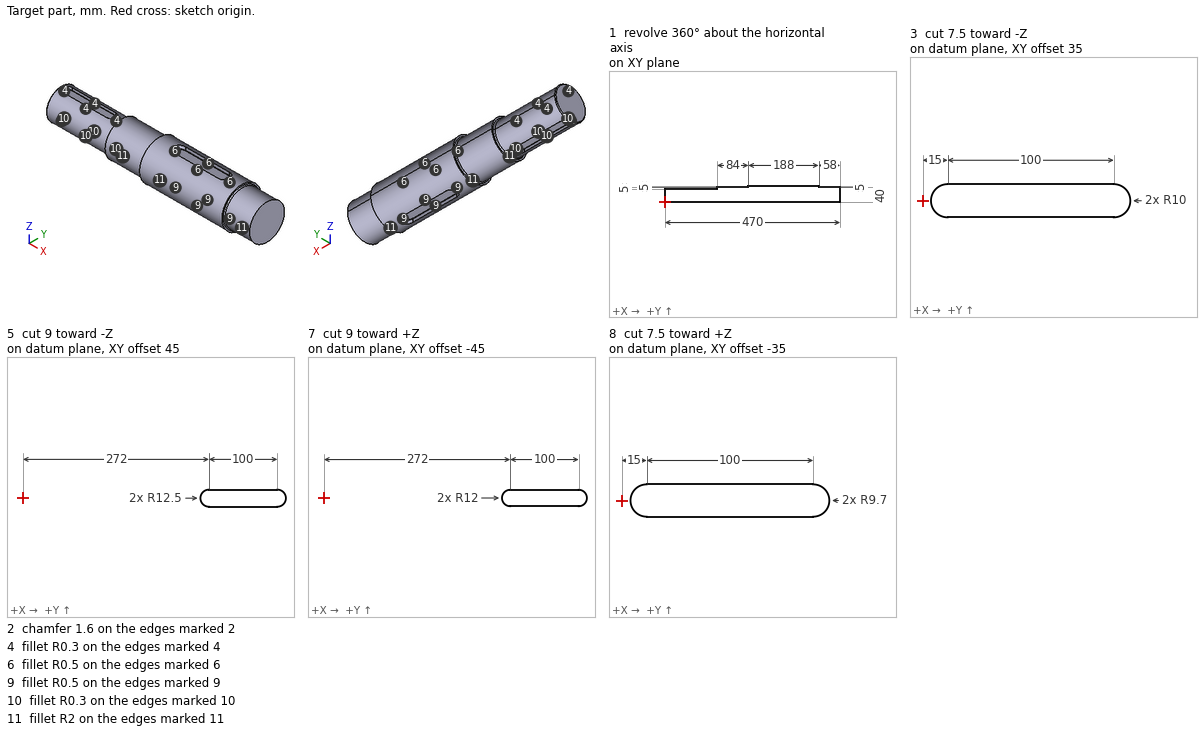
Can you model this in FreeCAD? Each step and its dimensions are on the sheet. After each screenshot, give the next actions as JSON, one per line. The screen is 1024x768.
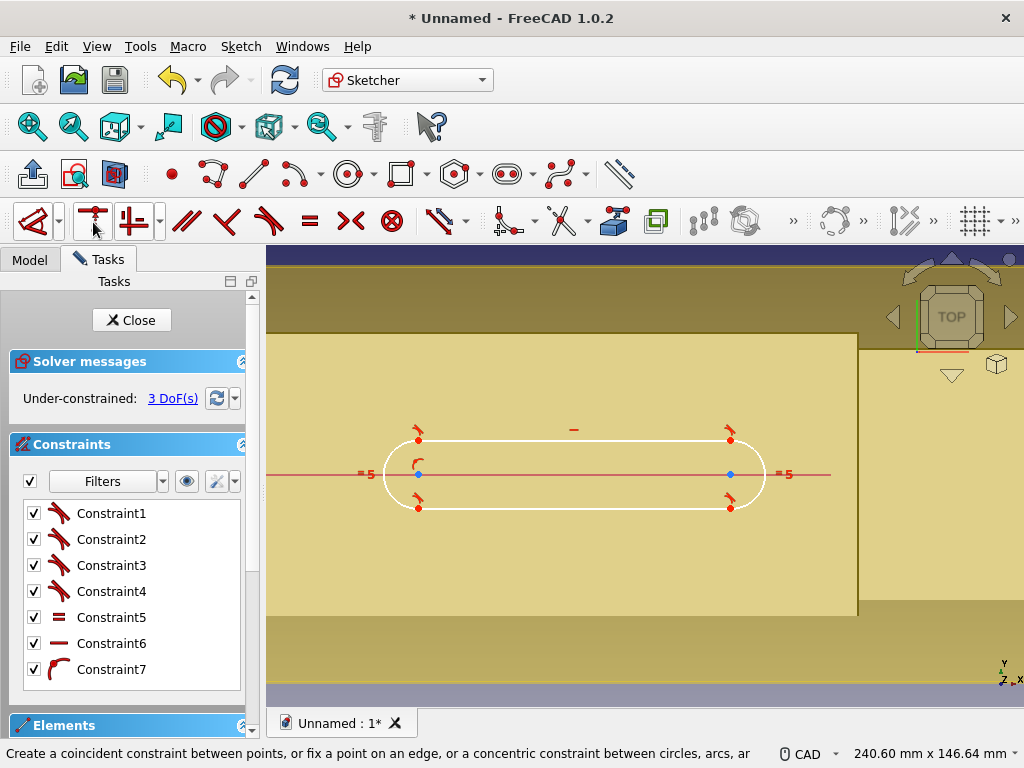
{"action": "left_click", "coordinate": [390, 455]}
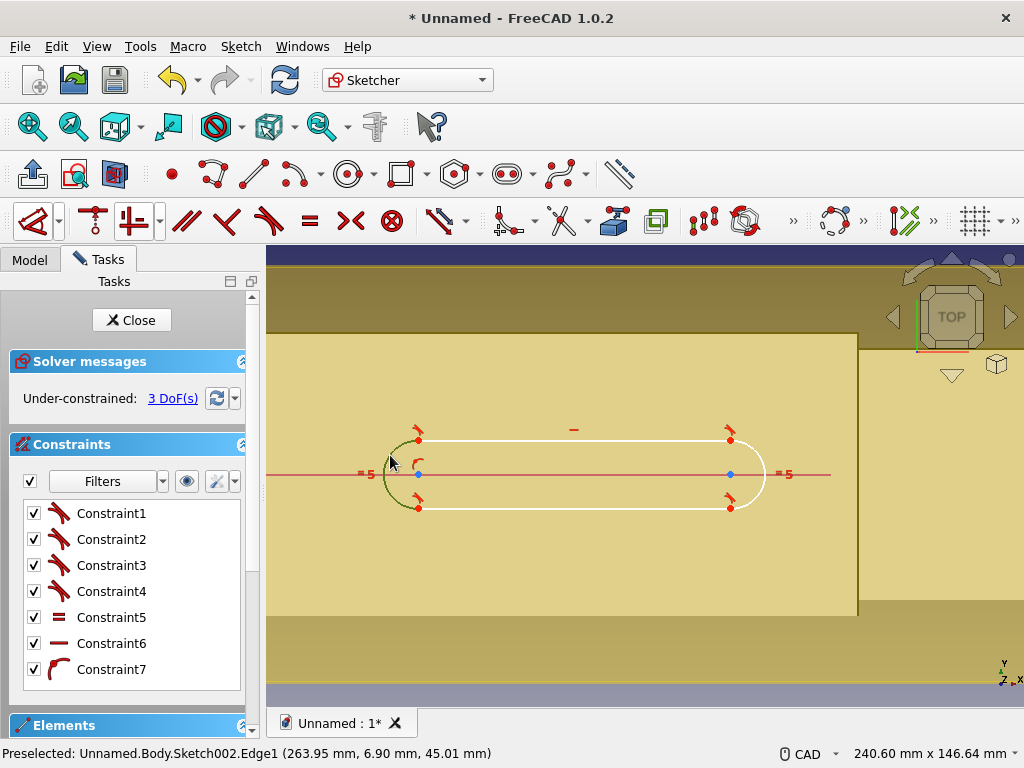
{"action": "left_click", "coordinate": [58, 222]}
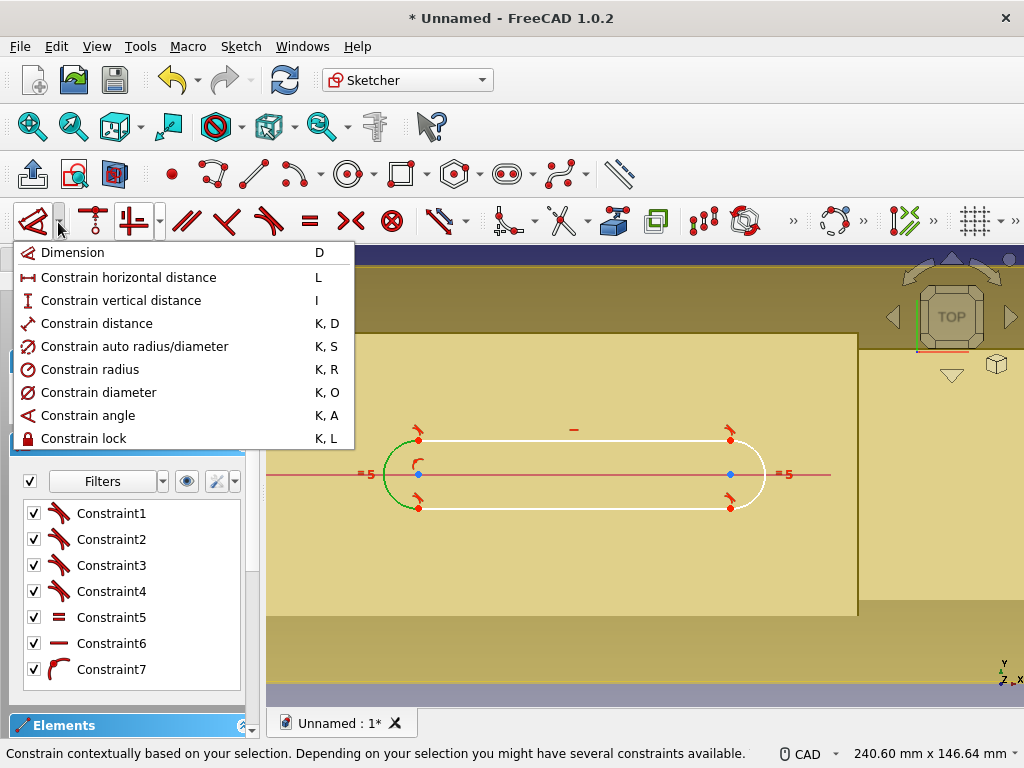
{"action": "left_click", "coordinate": [184, 370]}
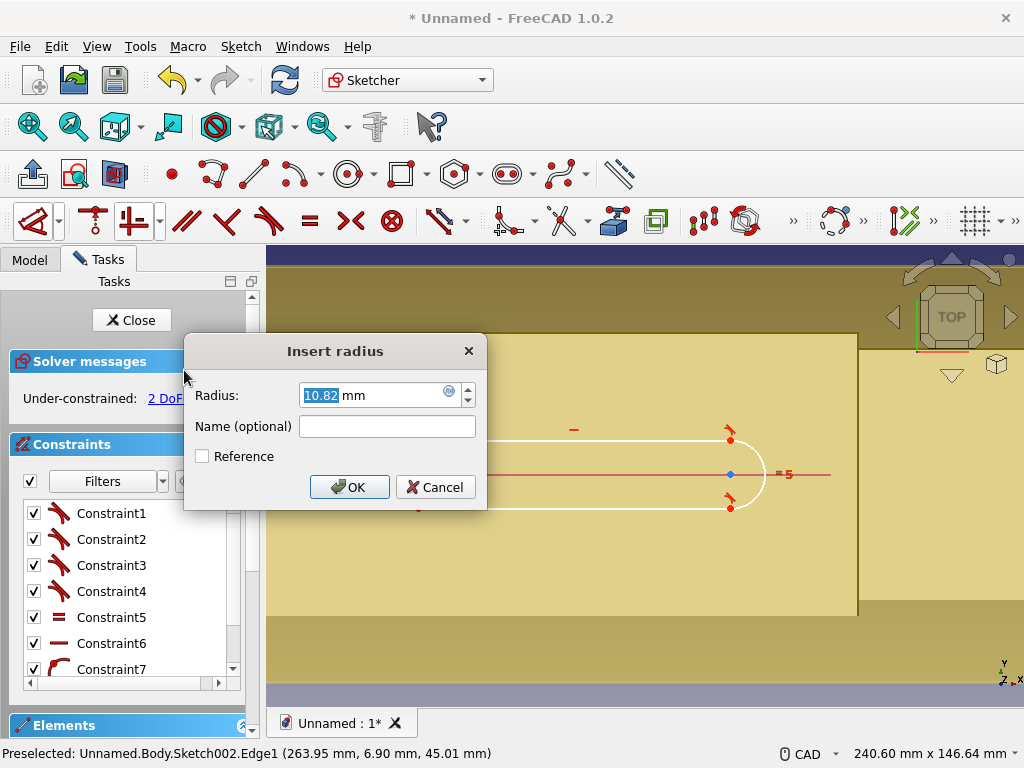
{"action": "type", "text": "12.5"}
{"action": "key", "text": "Return"}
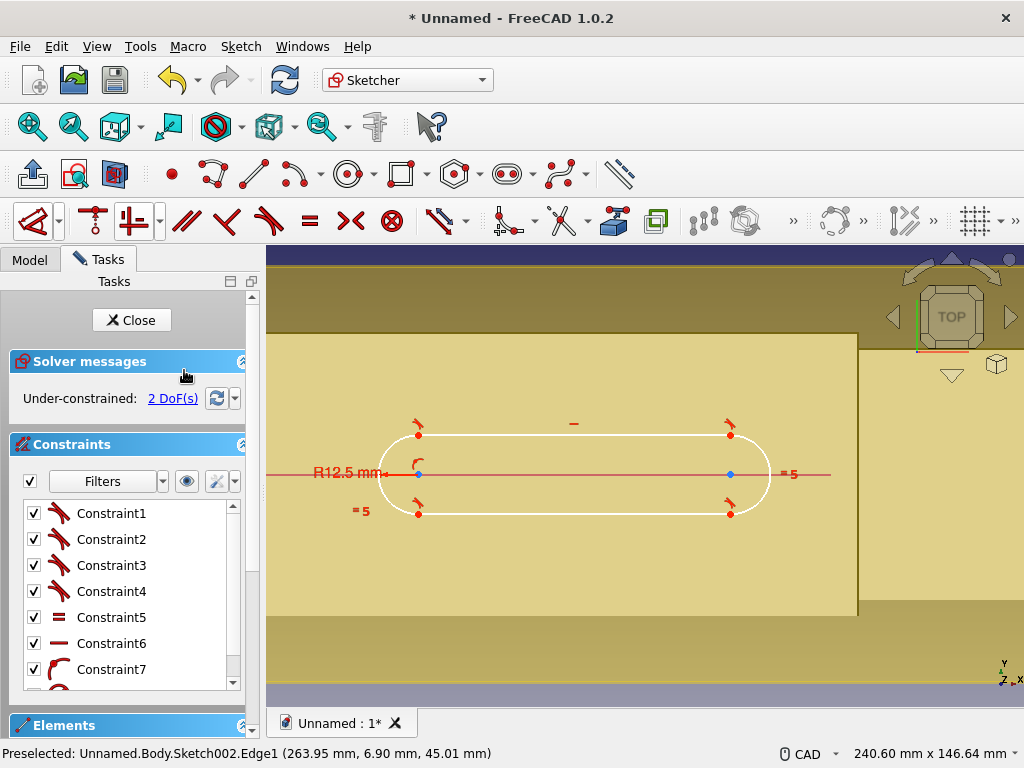
{"action": "left_click", "coordinate": [512, 435]}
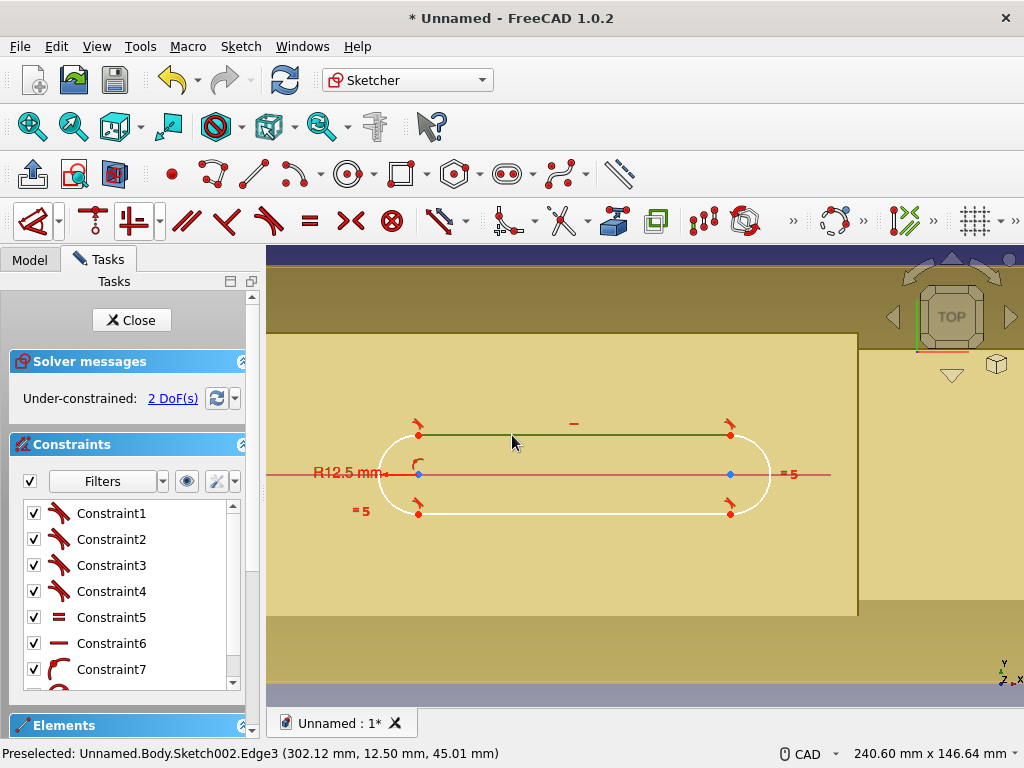
{"action": "key", "text": "l"}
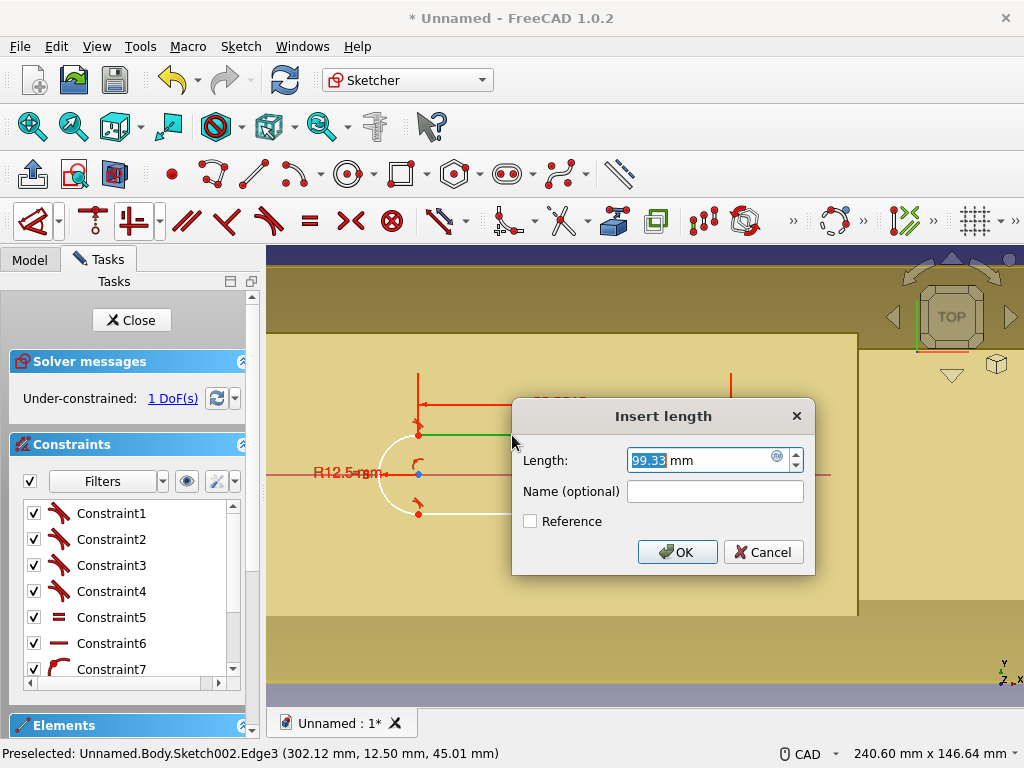
{"action": "type", "text": "100"}
{"action": "key", "text": "Return"}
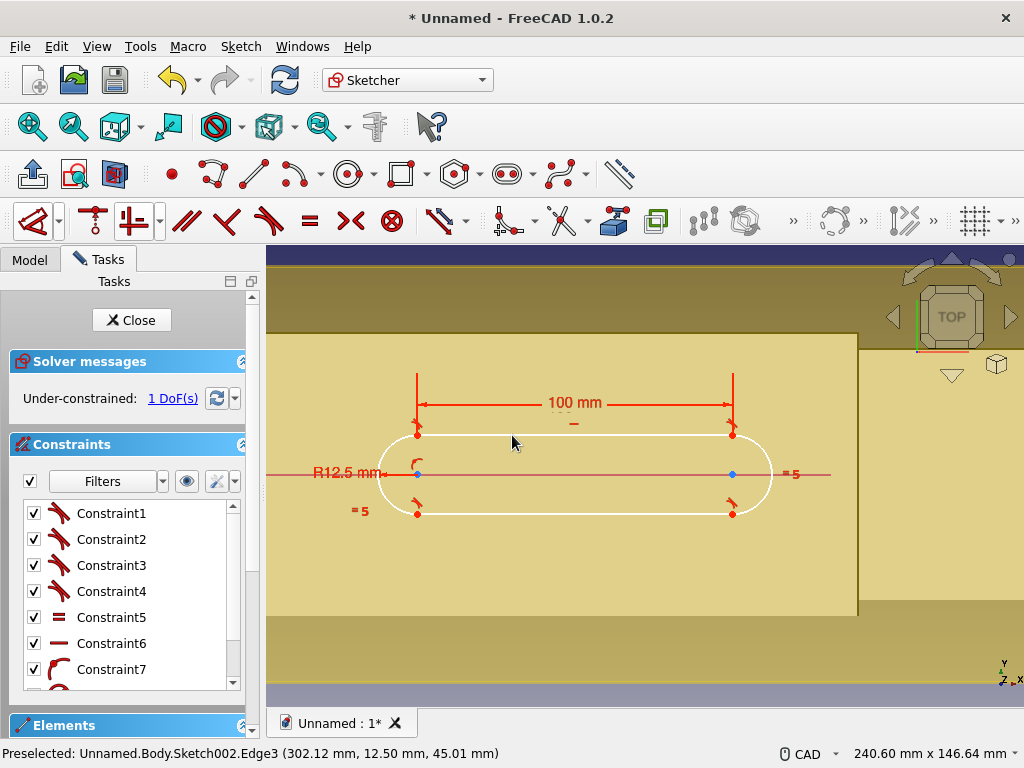
{"action": "left_click", "coordinate": [417, 435]}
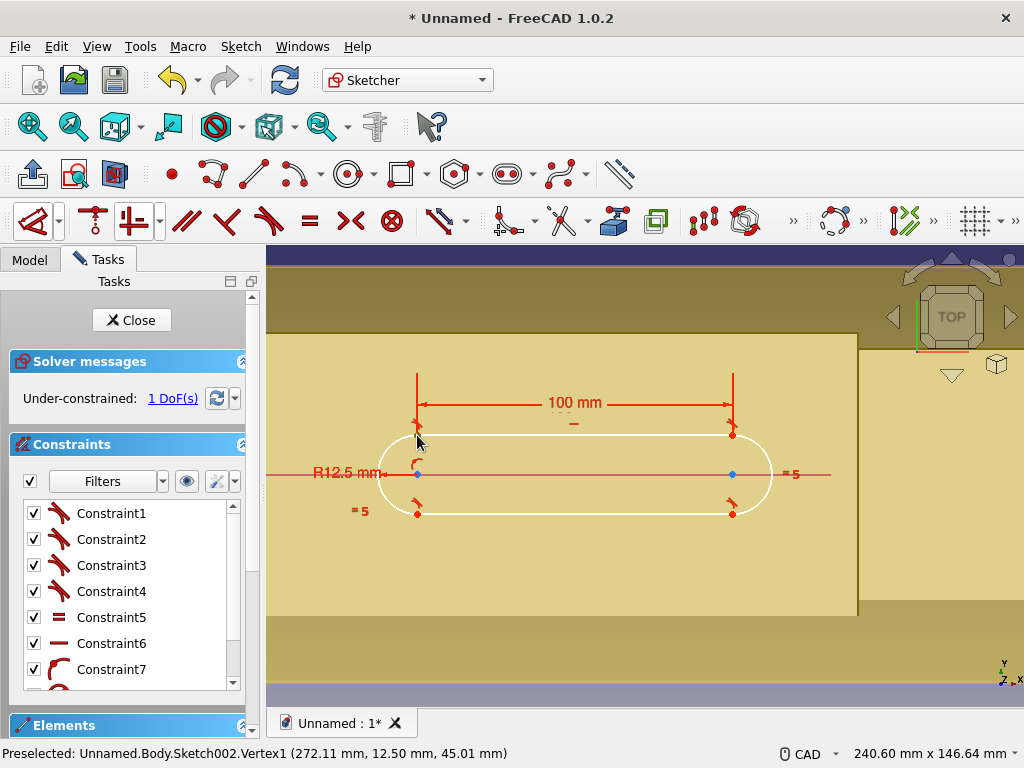
{"action": "key", "text": "l"}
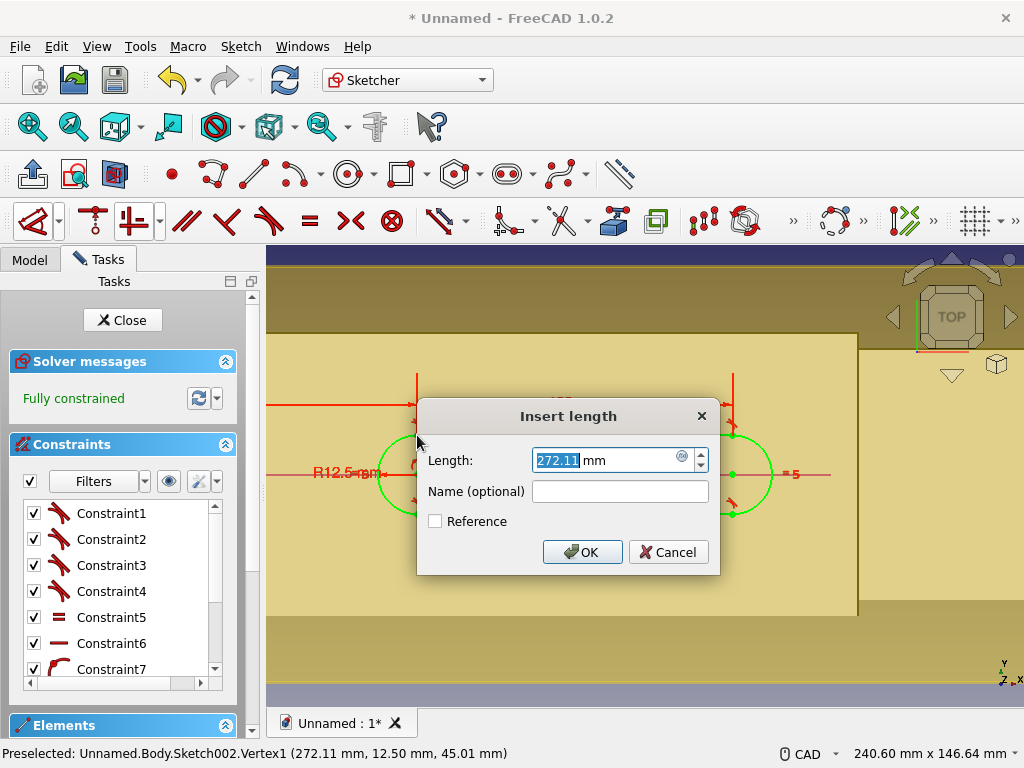
{"action": "type", "text": "272"}
{"action": "key", "text": "Return"}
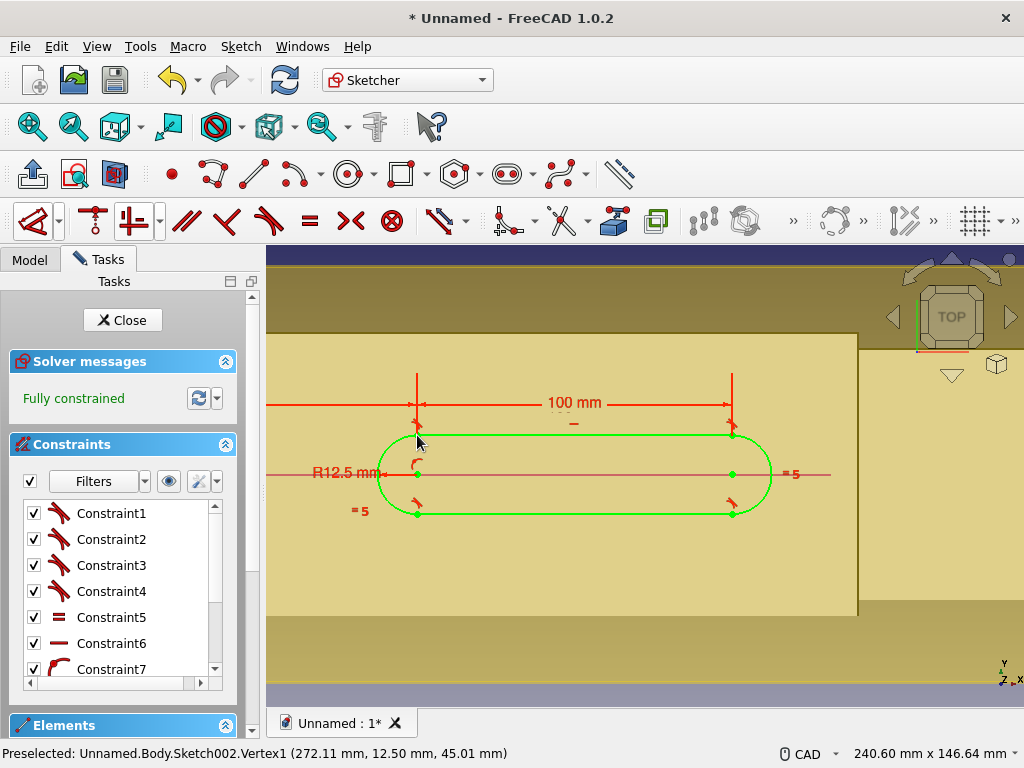
{"action": "left_click", "coordinate": [123, 320]}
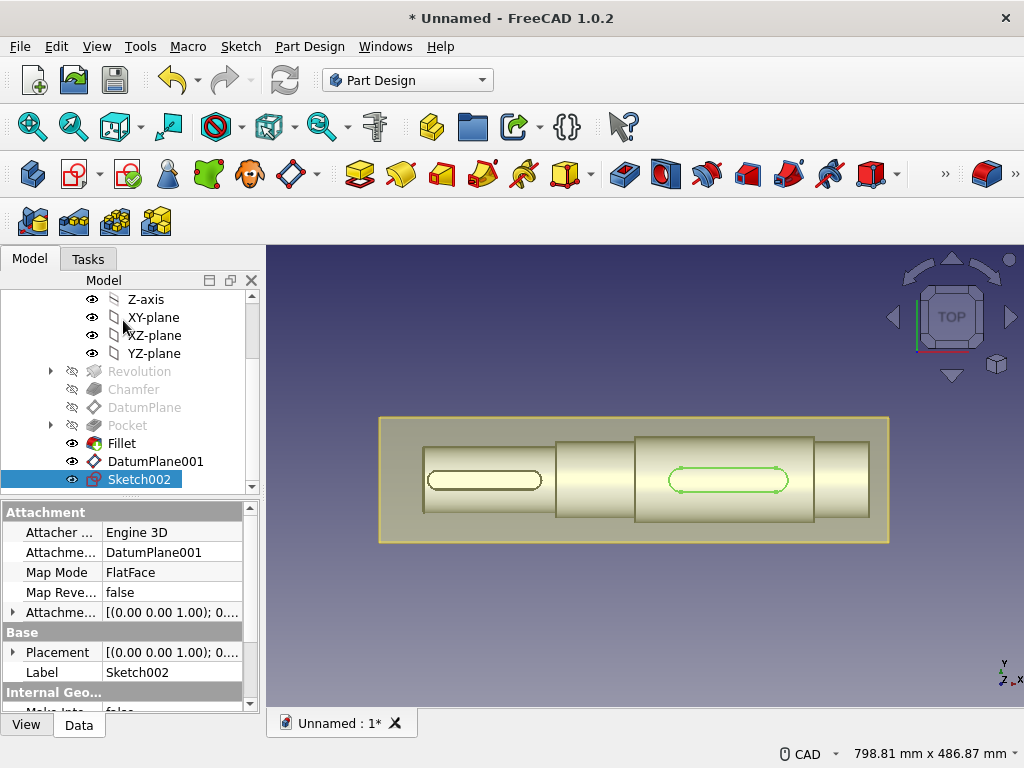
{"action": "left_click", "coordinate": [625, 174]}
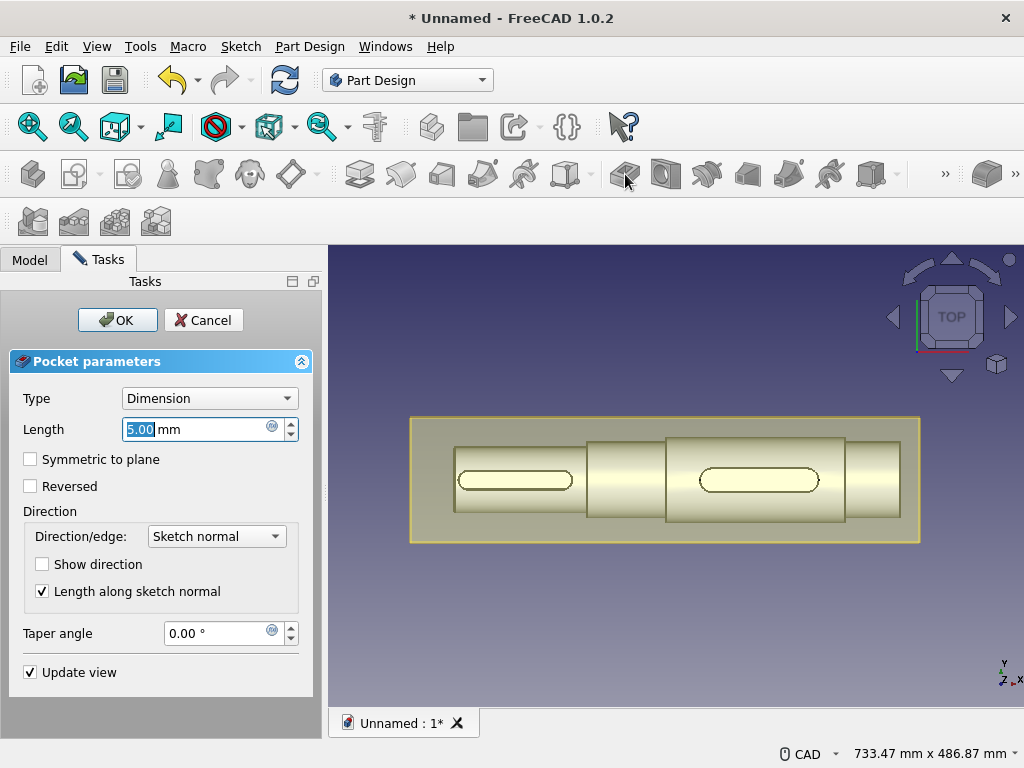
{"action": "type", "text": "9"}
{"action": "key", "text": "Tab"}